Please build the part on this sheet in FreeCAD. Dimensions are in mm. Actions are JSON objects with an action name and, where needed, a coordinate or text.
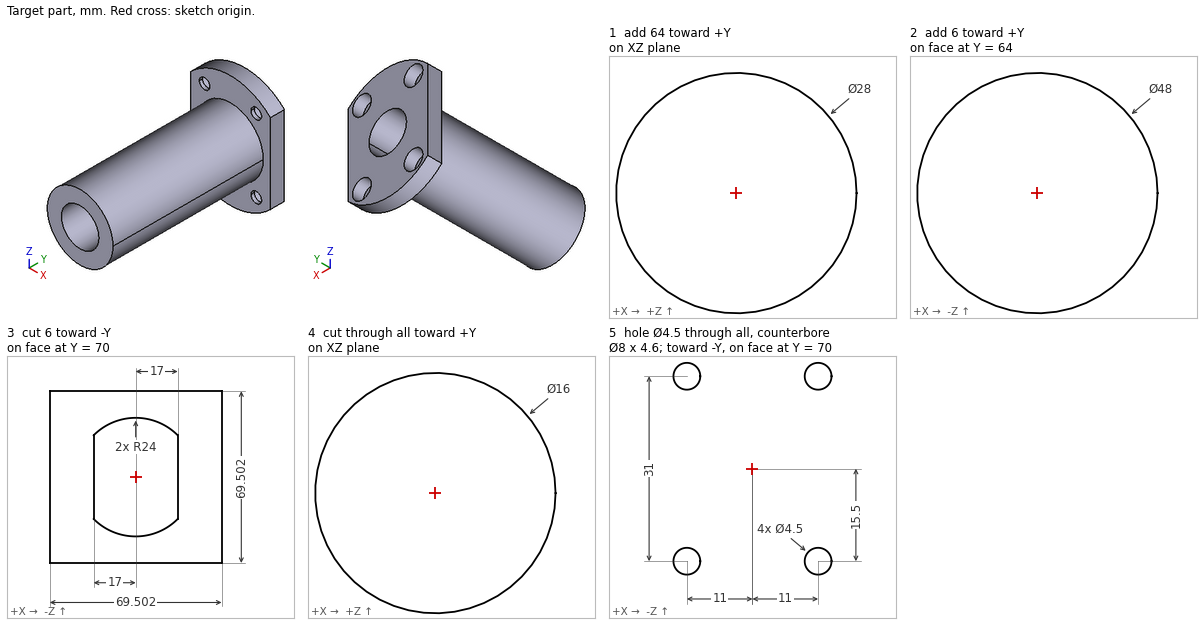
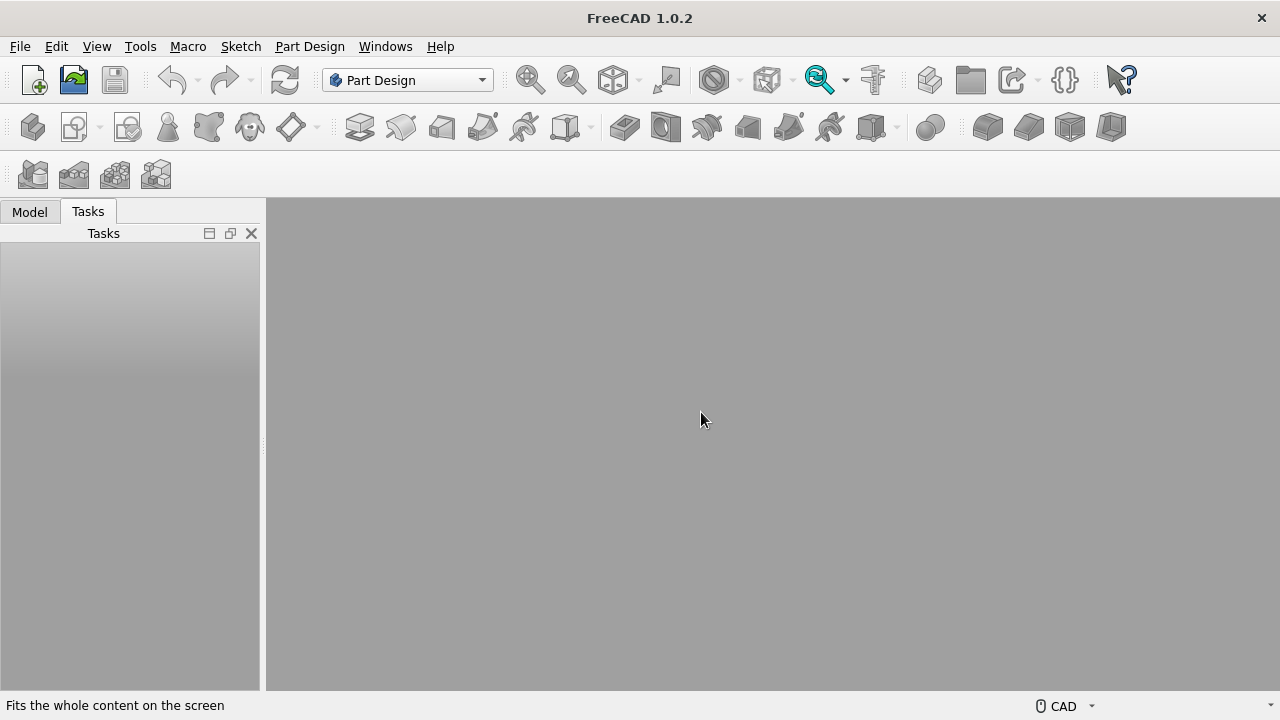
{"action": "left_click", "coordinate": [33, 80]}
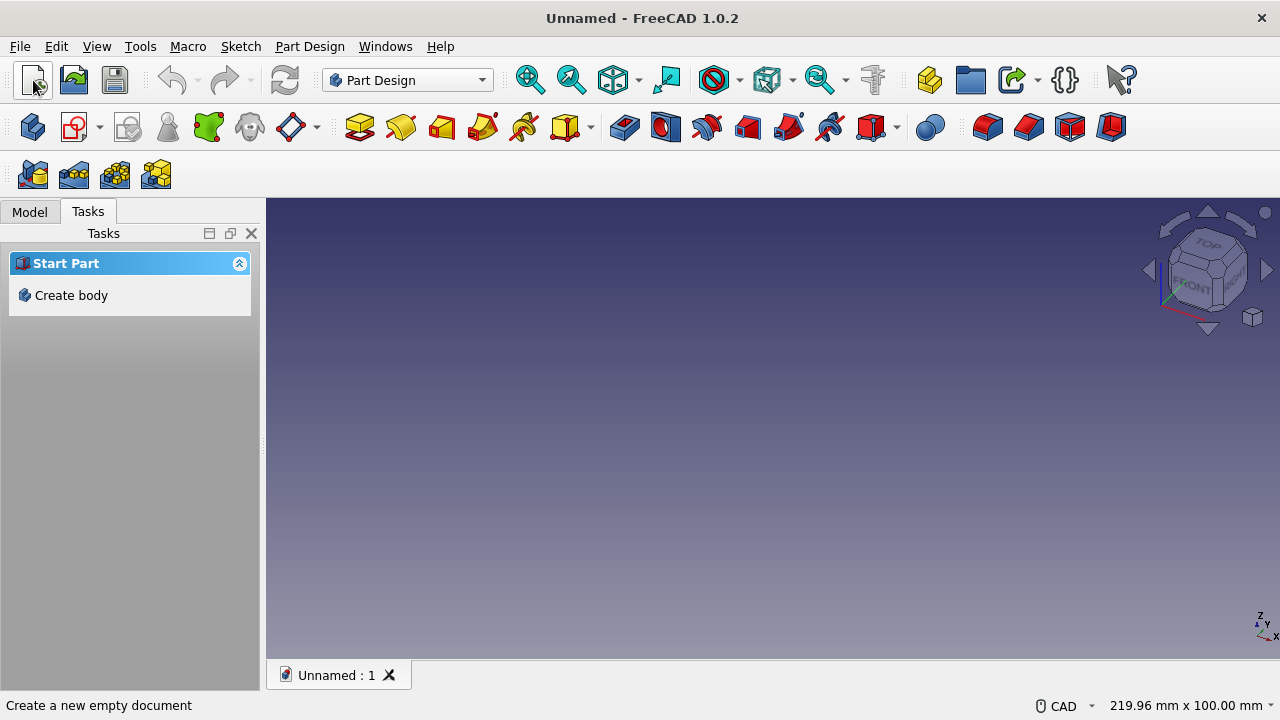
{"action": "left_click", "coordinate": [74, 128]}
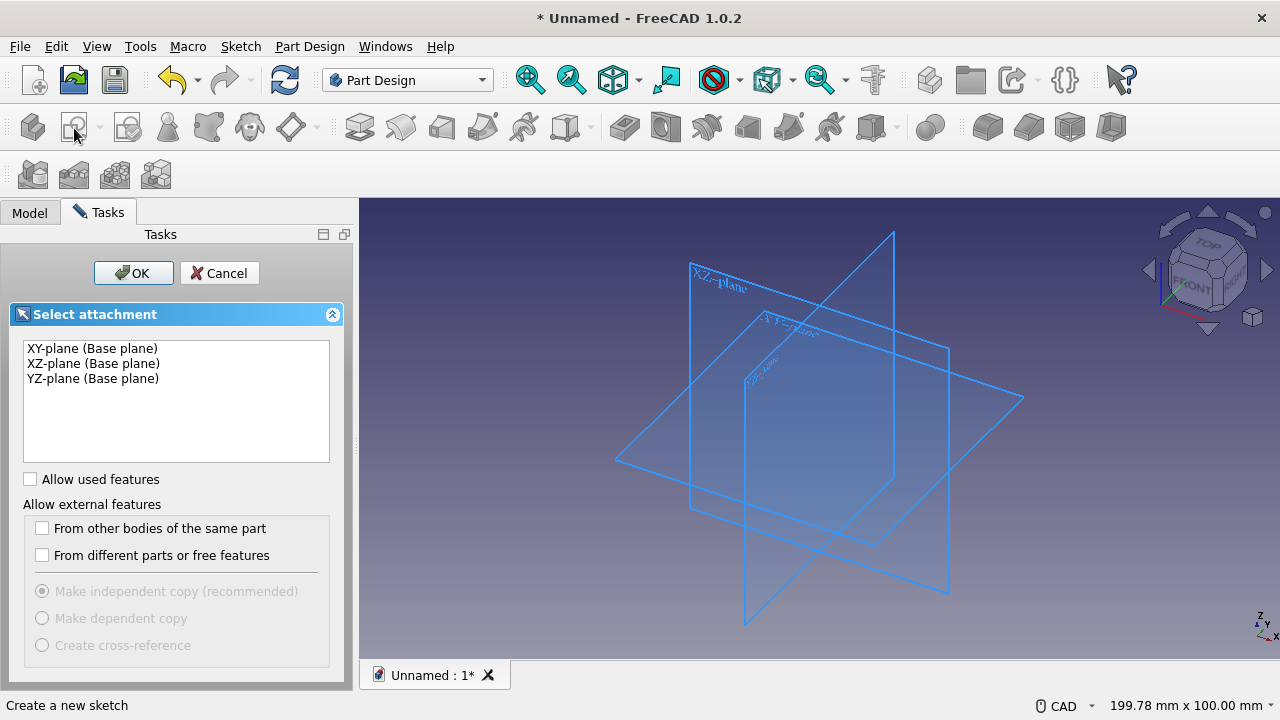
{"action": "left_click", "coordinate": [84, 364]}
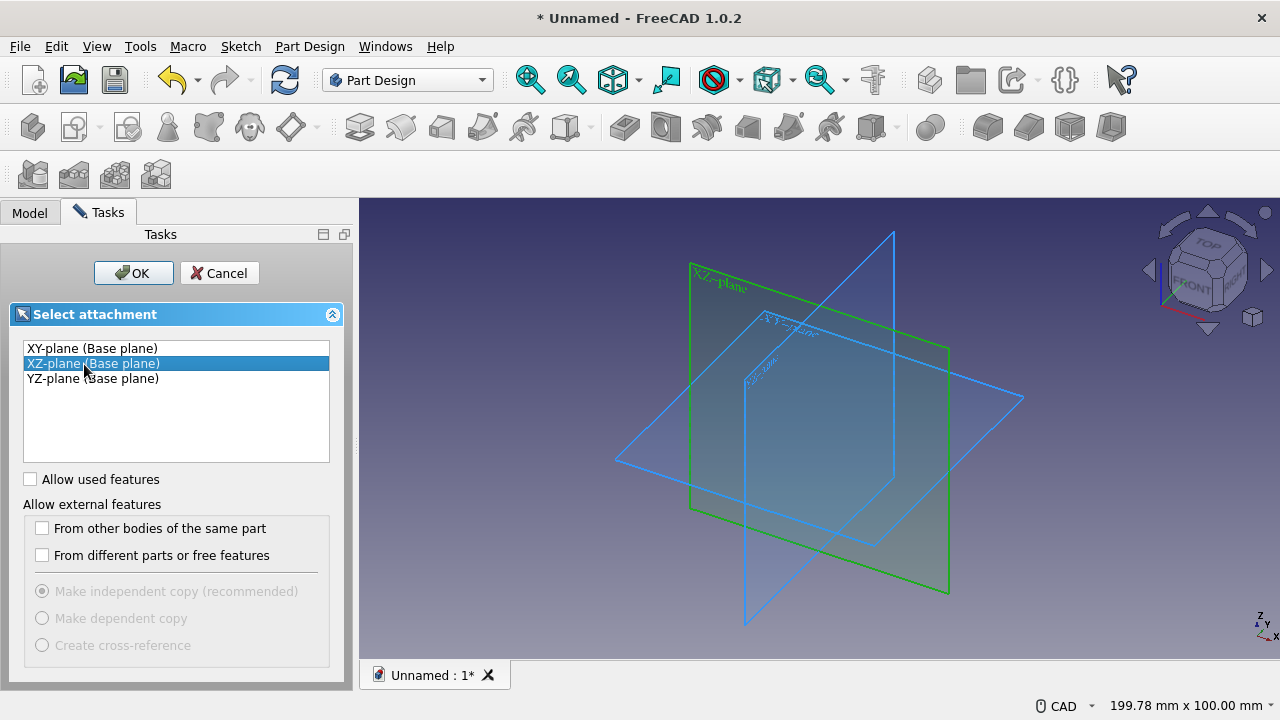
{"action": "left_click", "coordinate": [134, 273]}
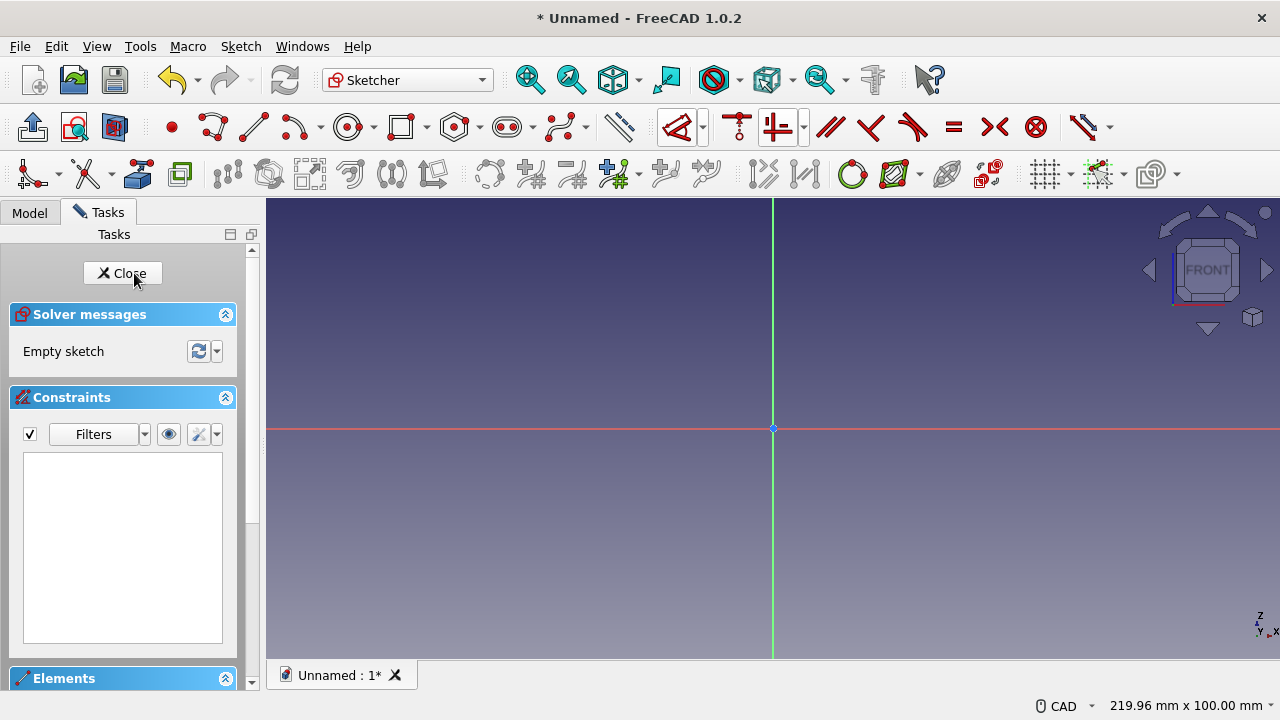
{"action": "scroll", "coordinate": [829, 428], "scroll_direction": "up", "scroll_amount": 4}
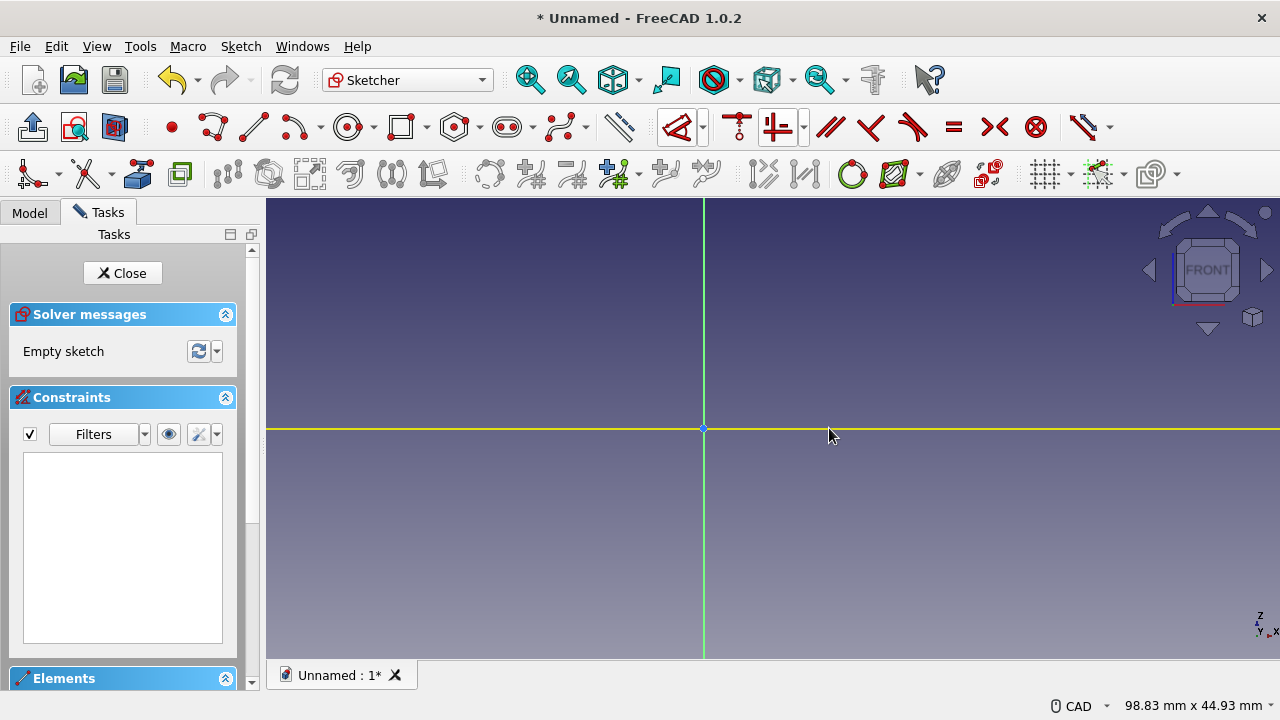
{"action": "left_click", "coordinate": [348, 128]}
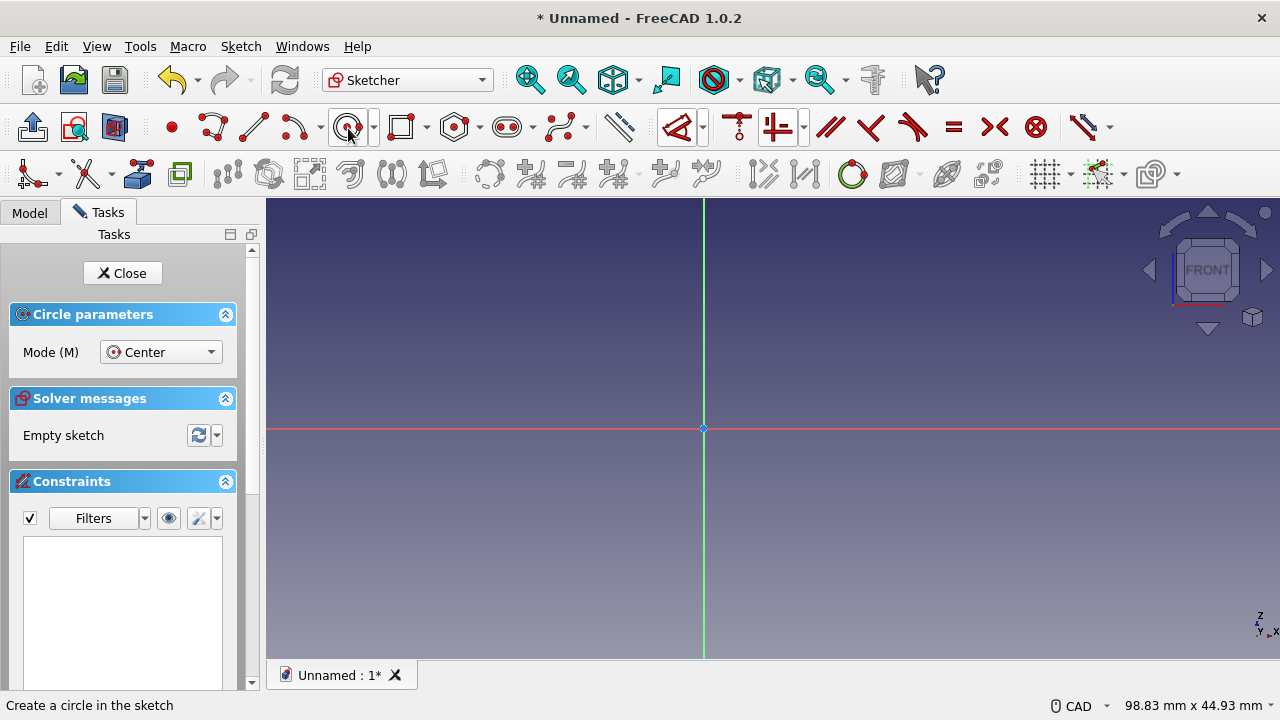
{"action": "left_click", "coordinate": [704, 428]}
{"action": "left_click", "coordinate": [805, 327]}
{"action": "key", "text": "Escape"}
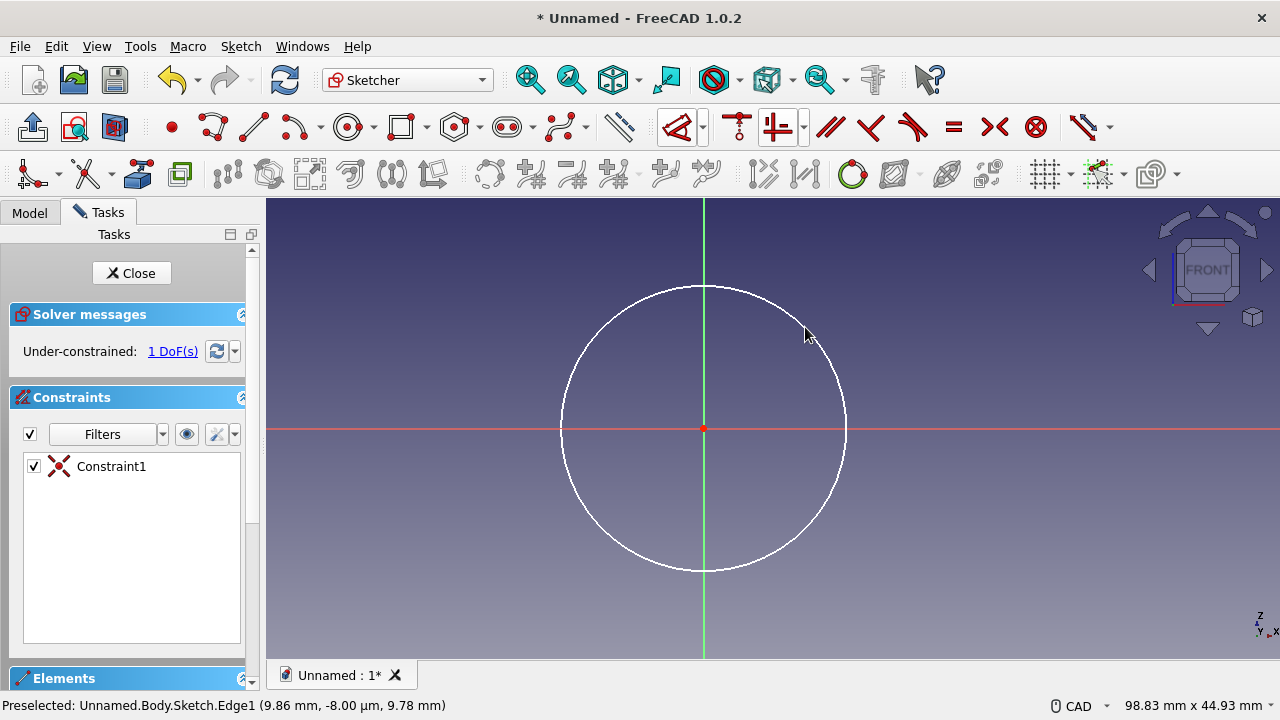
{"action": "left_click", "coordinate": [804, 327]}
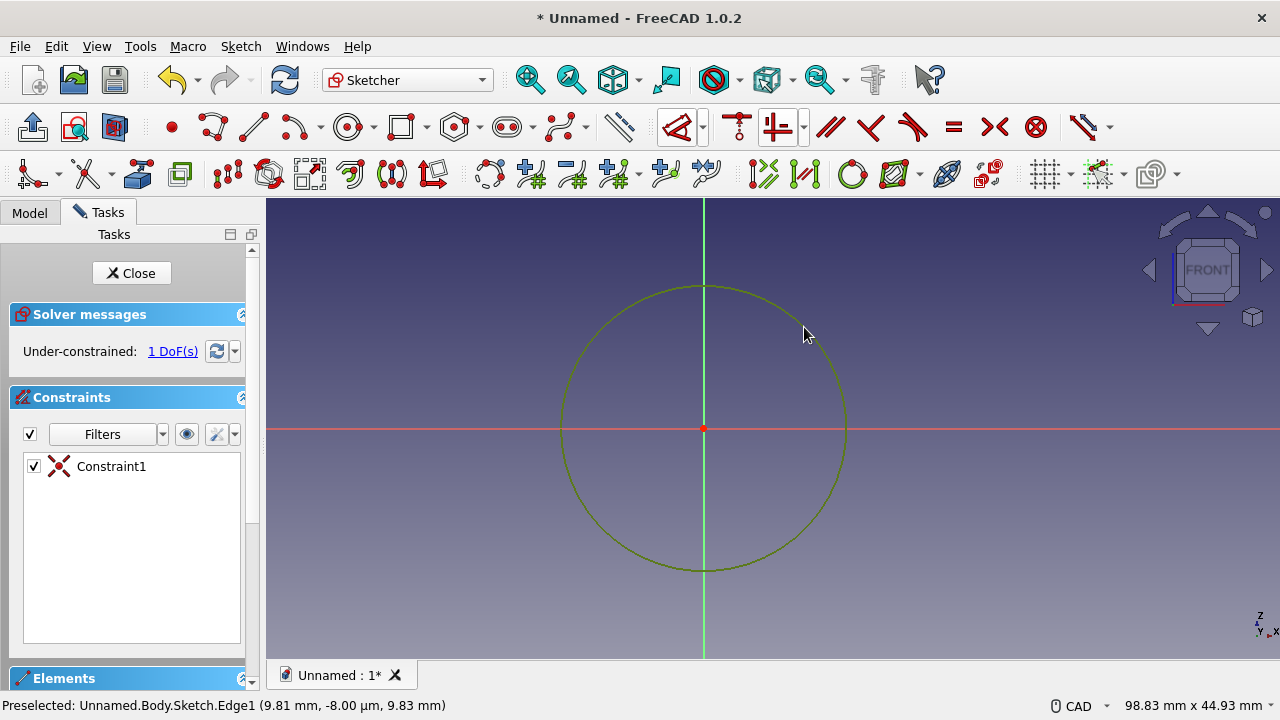
{"action": "left_click", "coordinate": [702, 128]}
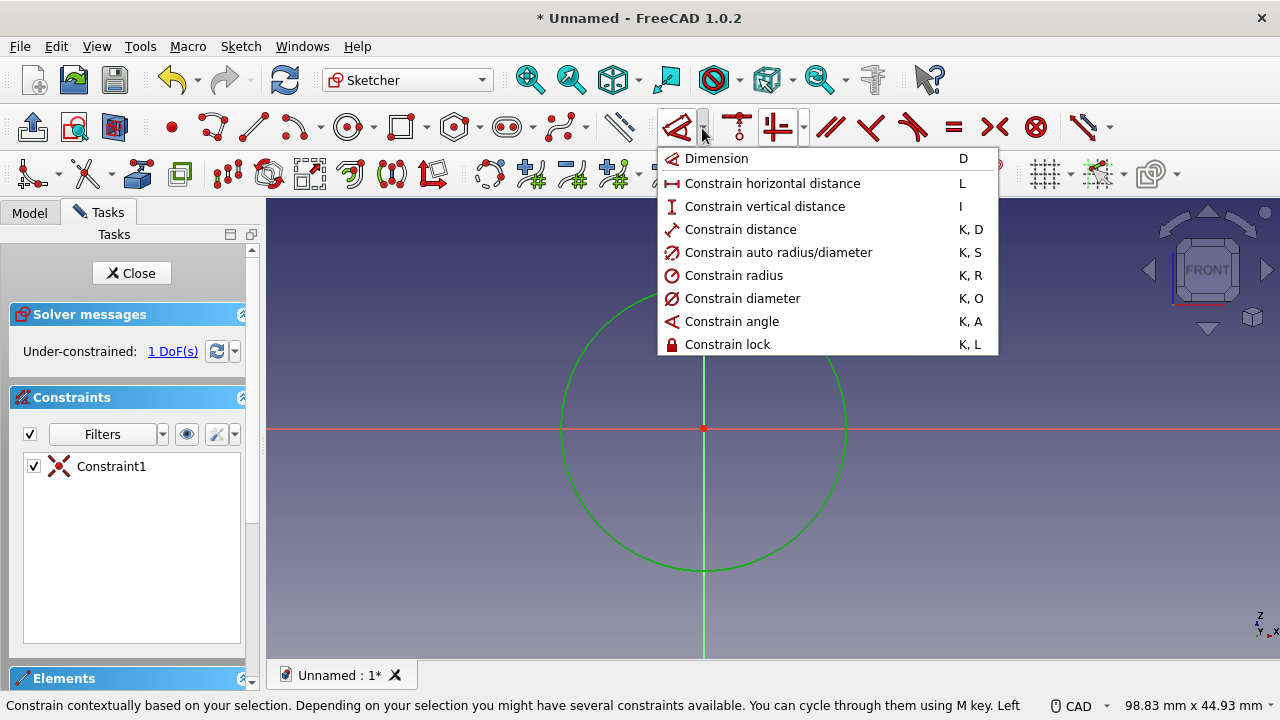
{"action": "left_click", "coordinate": [828, 298]}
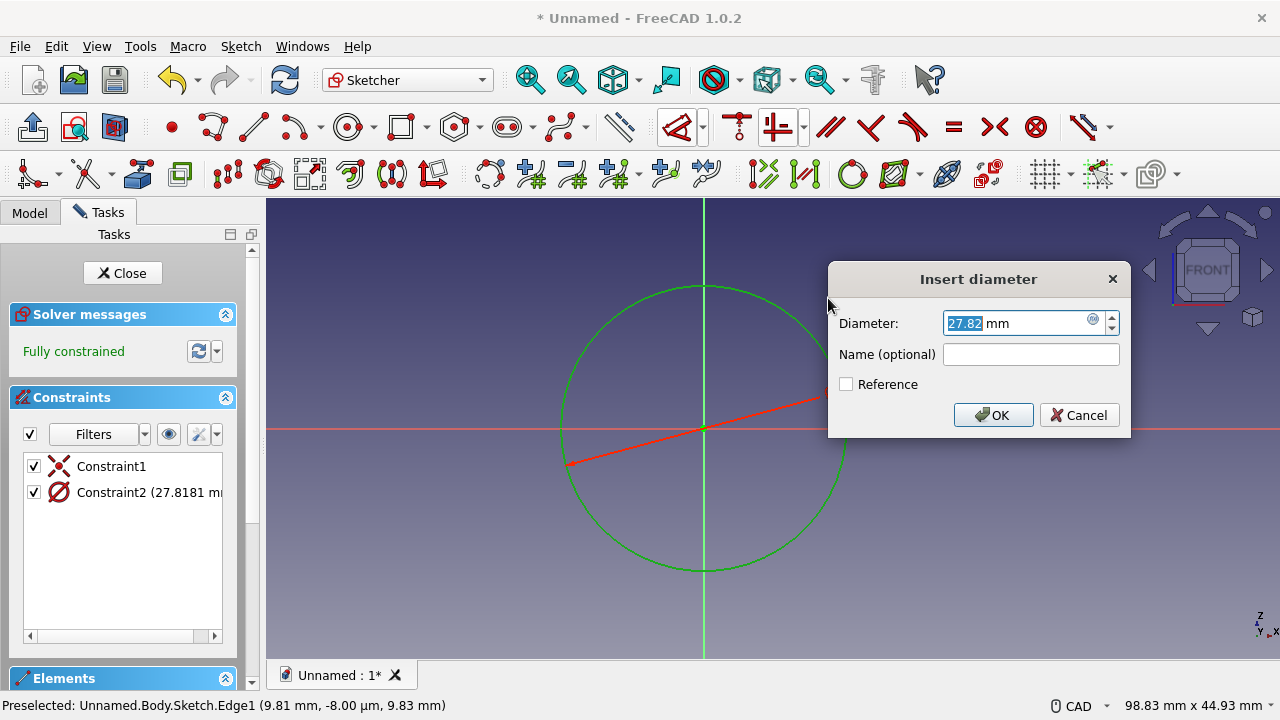
{"action": "type", "text": "28"}
{"action": "key", "text": "Return"}